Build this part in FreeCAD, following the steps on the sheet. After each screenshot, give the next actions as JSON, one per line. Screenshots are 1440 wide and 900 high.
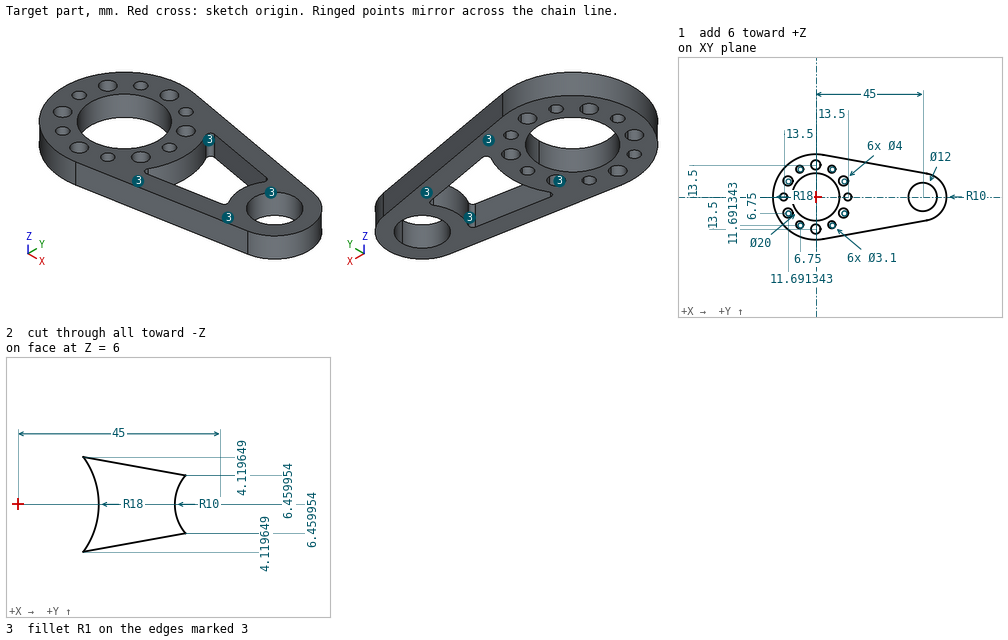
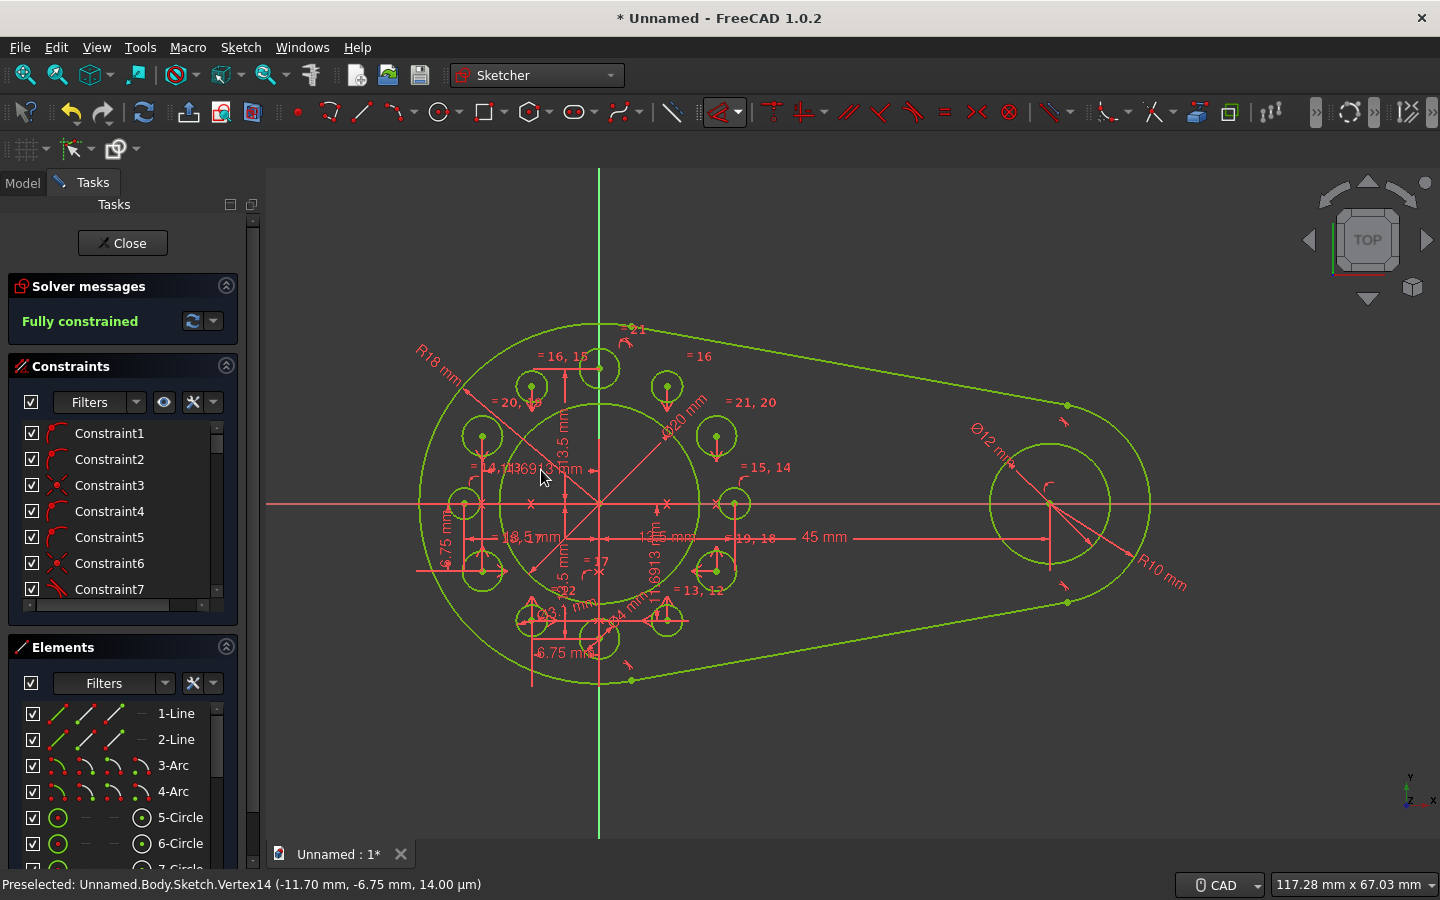
{"action": "left_click", "coordinate": [123, 243]}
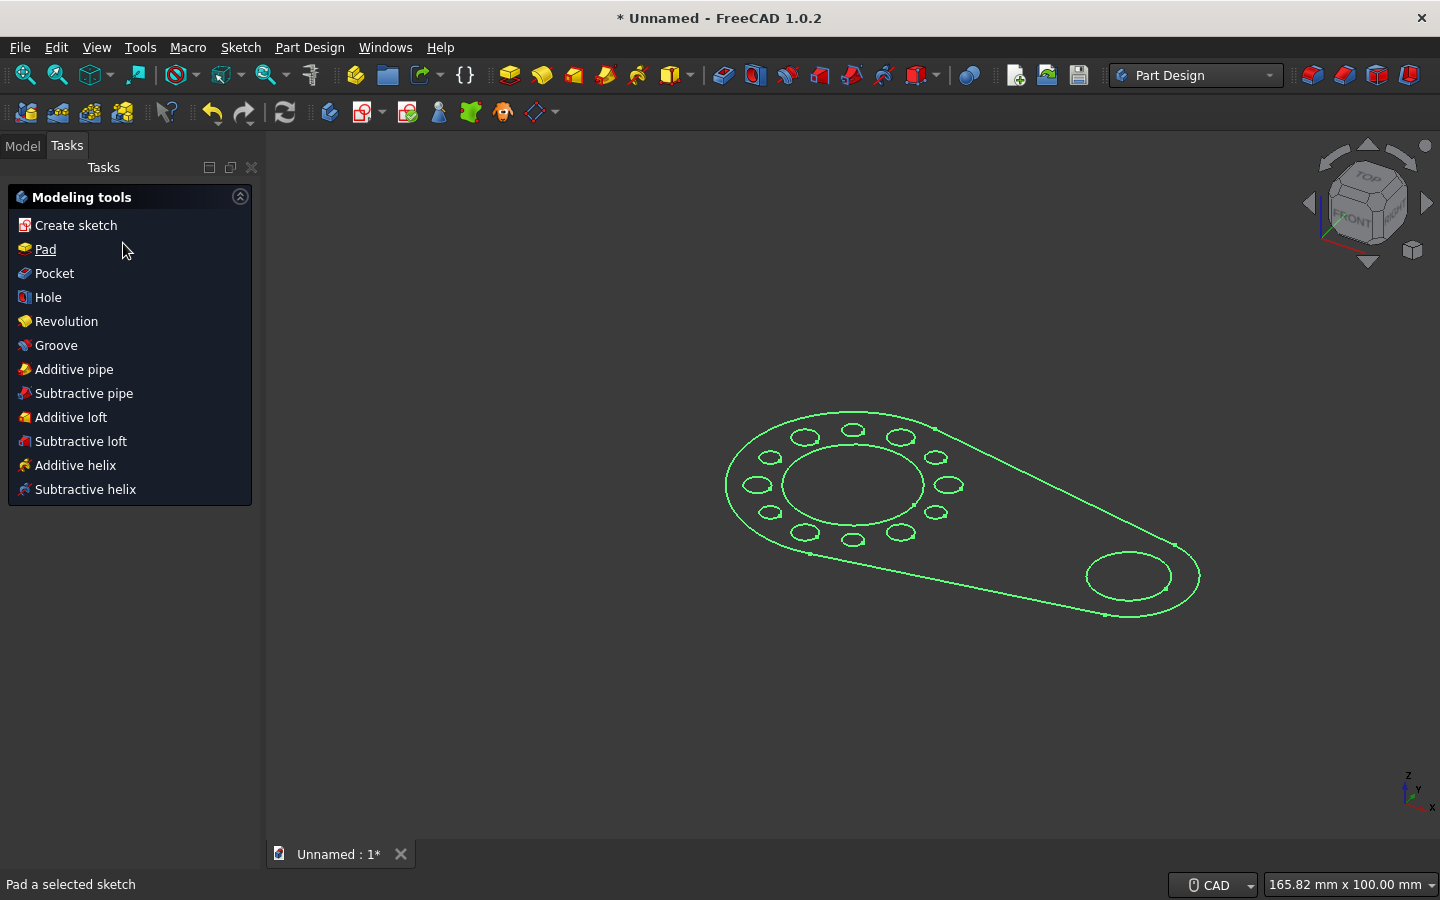
{"action": "left_click", "coordinate": [510, 76]}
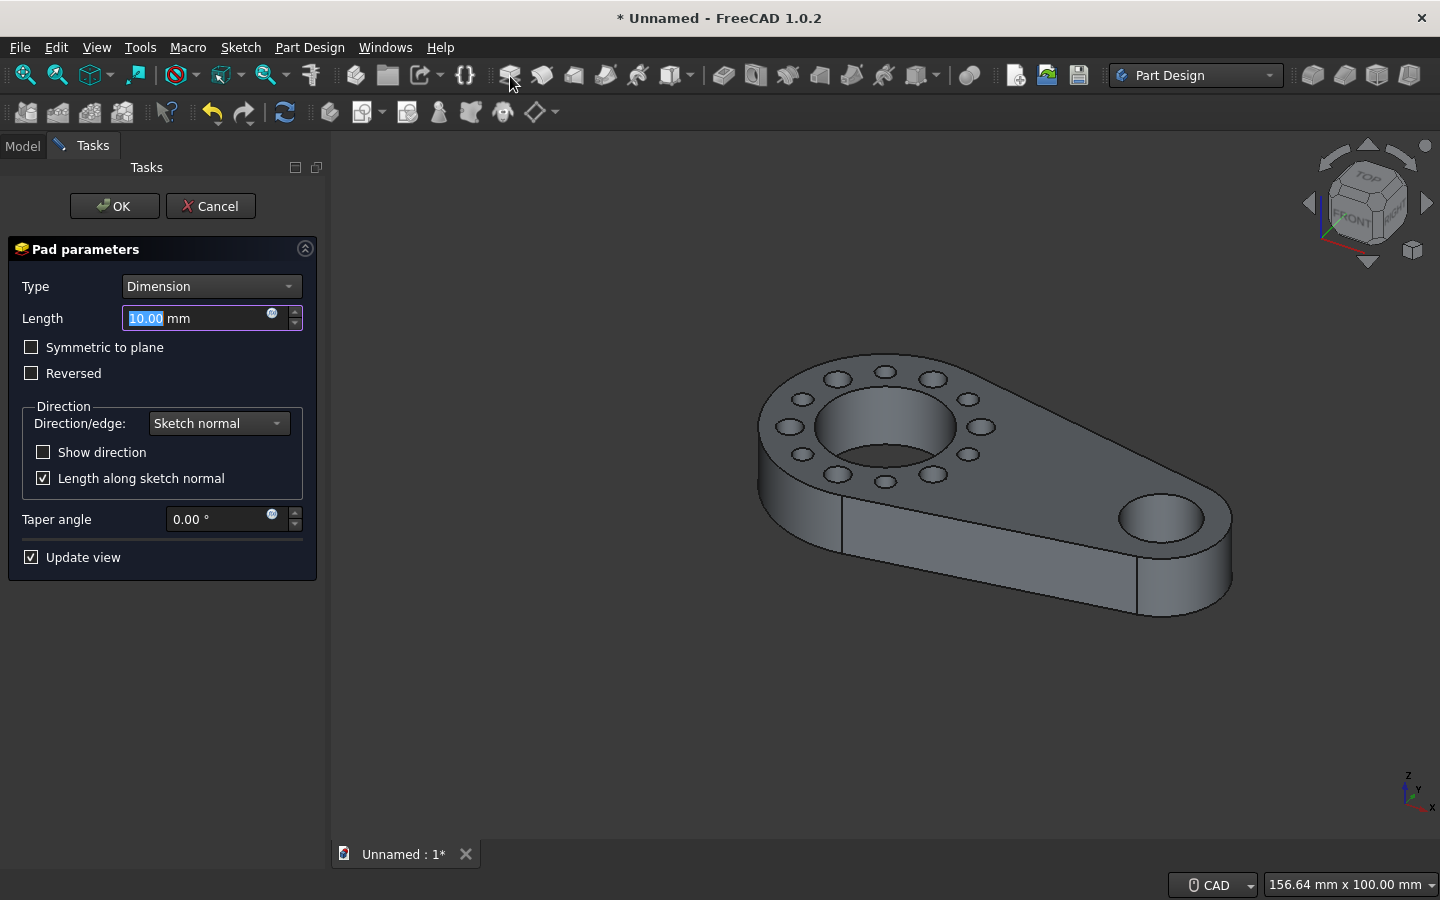
{"action": "type", "text": "6"}
{"action": "key", "text": "Tab"}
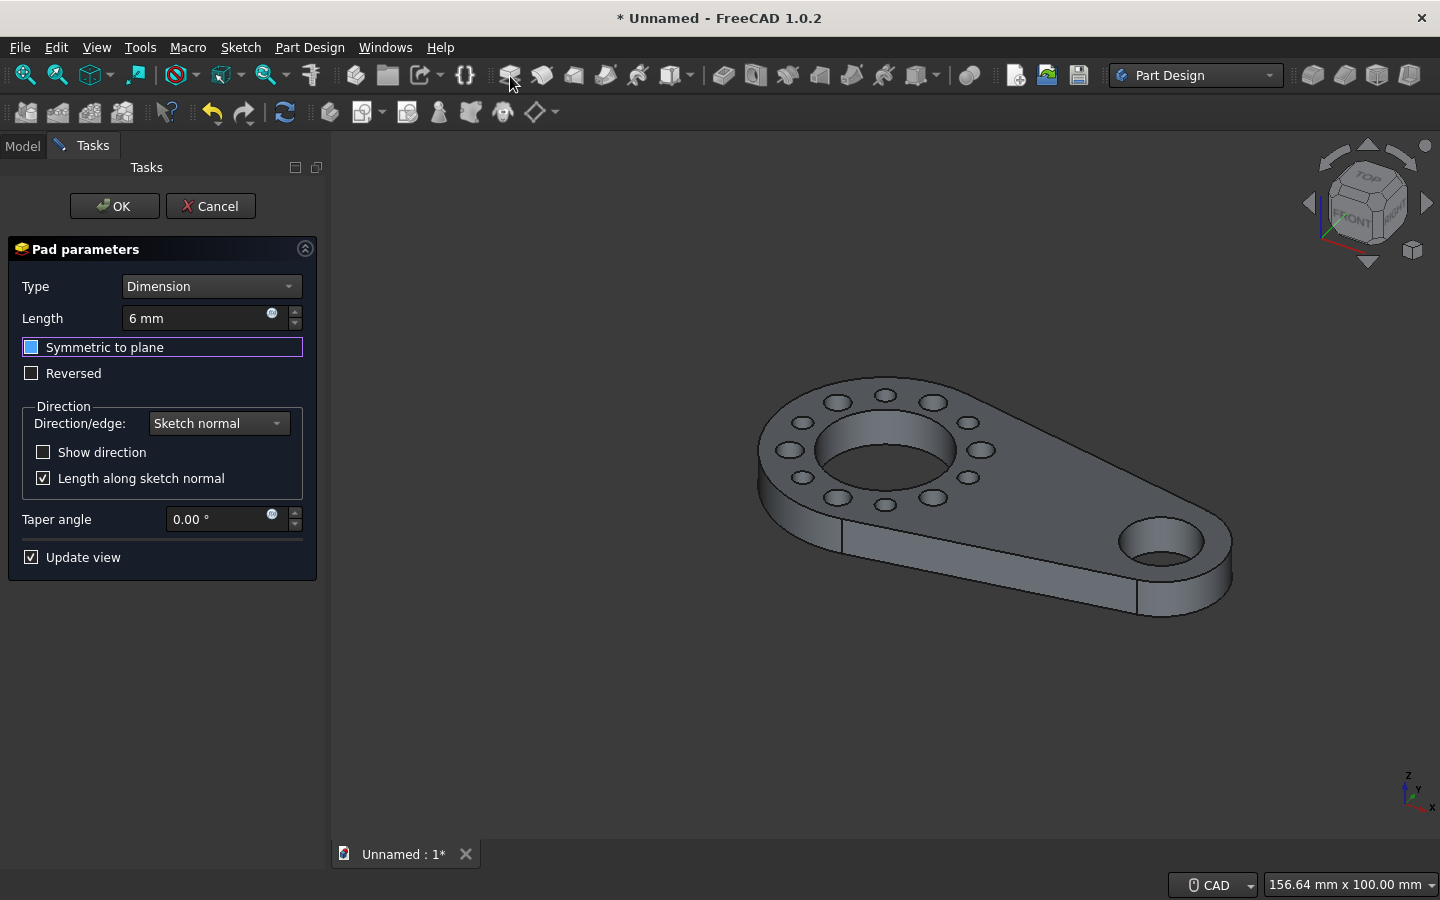
{"action": "left_click", "coordinate": [115, 206]}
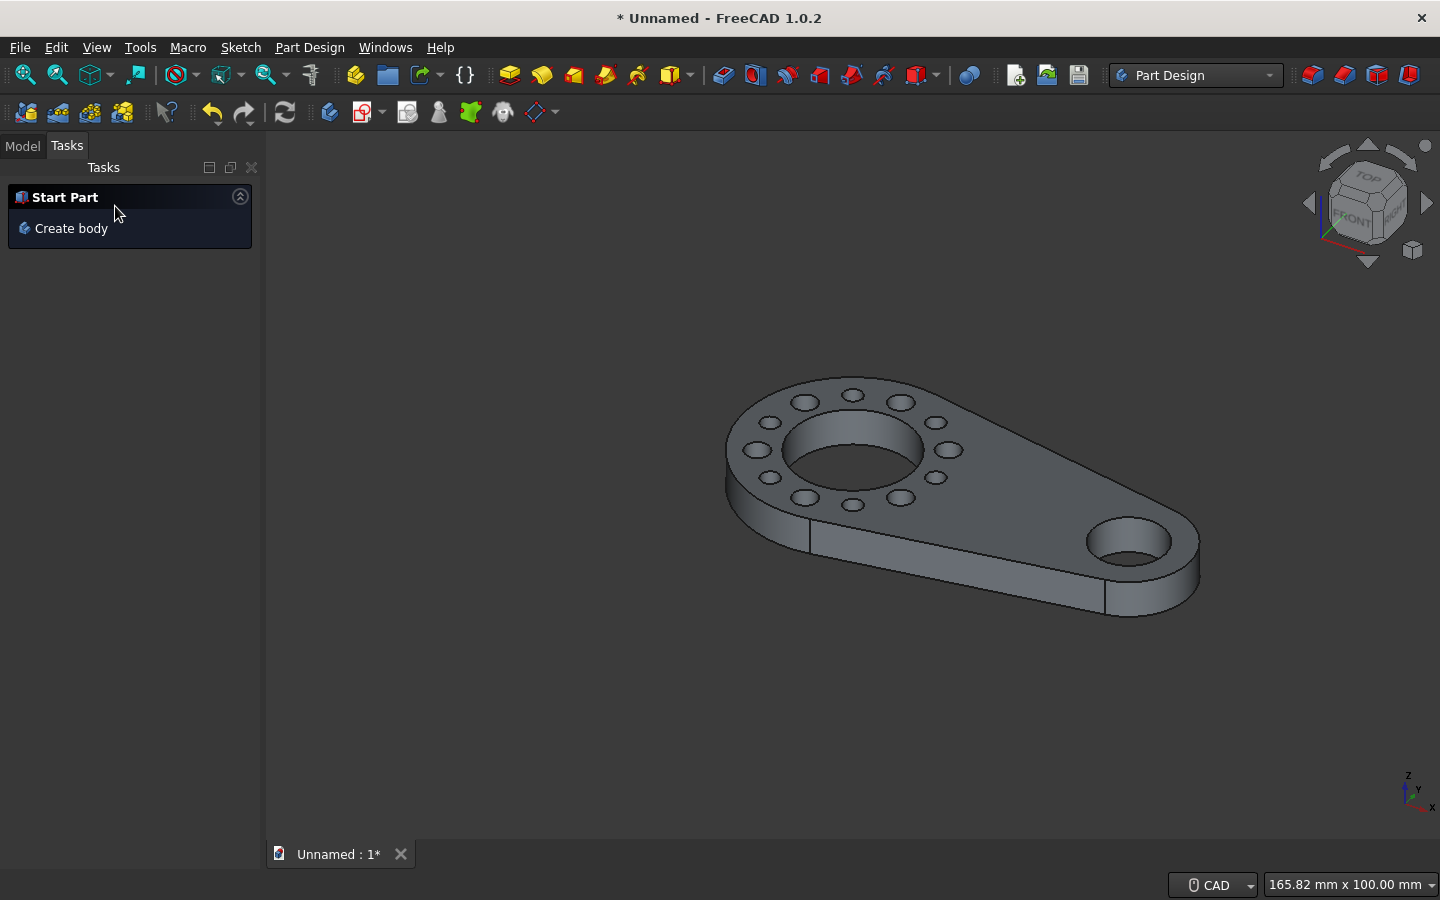
{"action": "left_click", "coordinate": [1030, 508]}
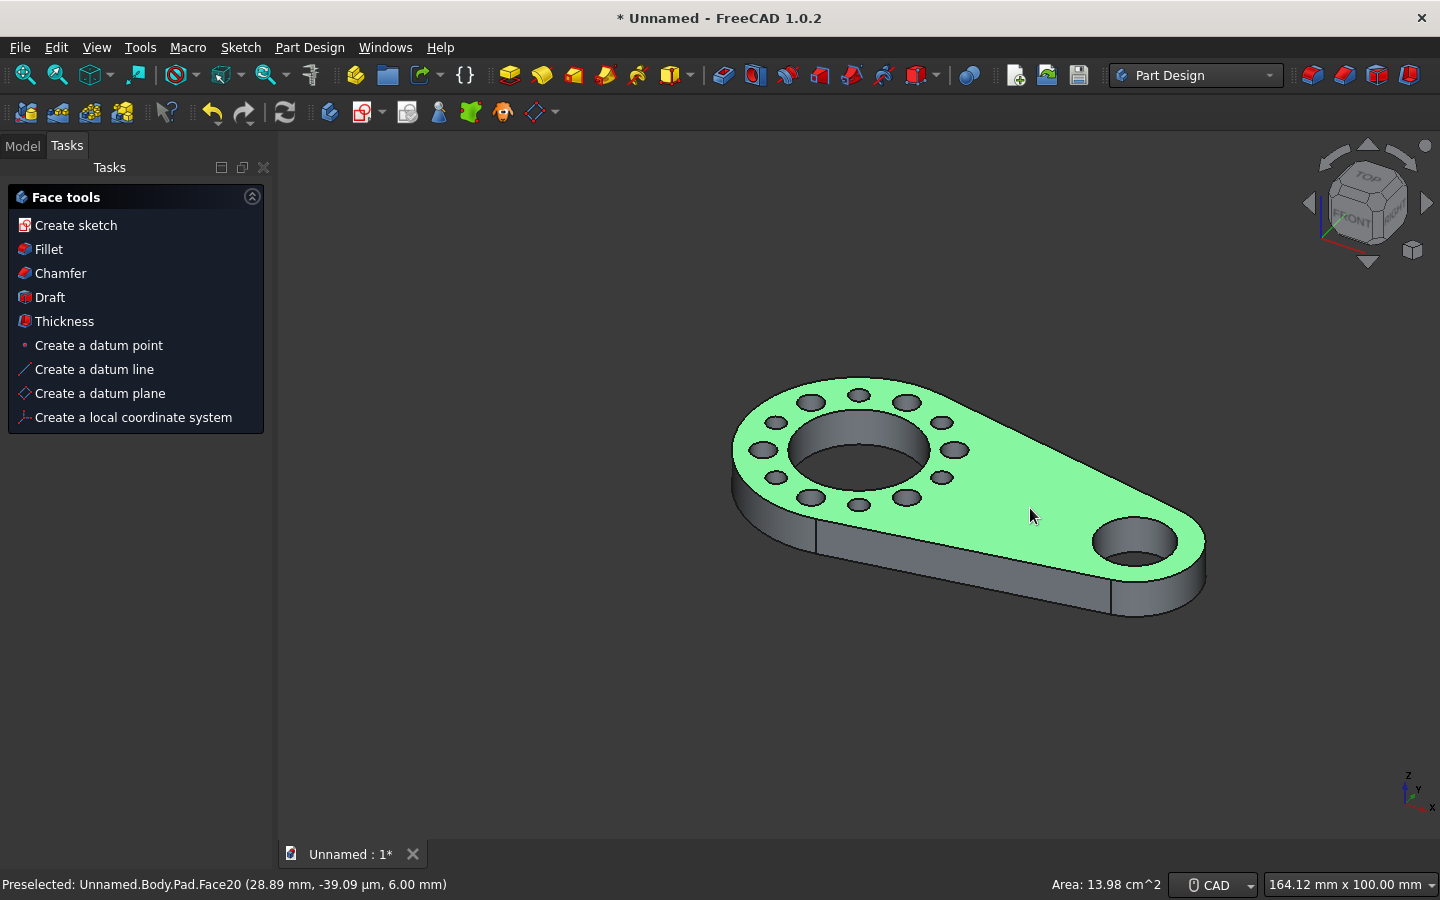
{"action": "left_click", "coordinate": [362, 112]}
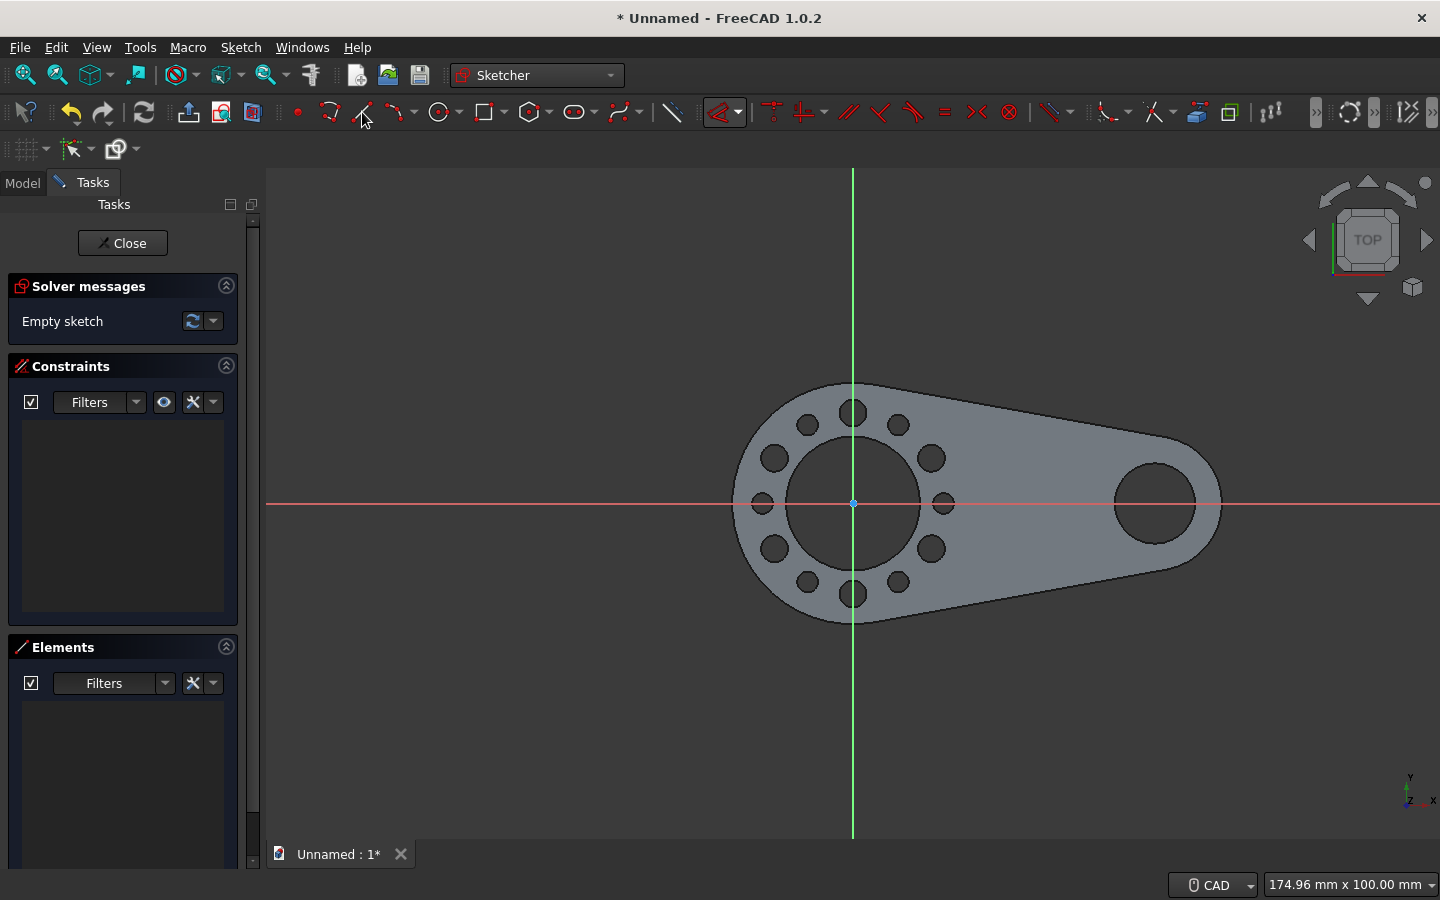
{"action": "scroll", "coordinate": [1091, 504], "scroll_direction": "up", "scroll_amount": 5}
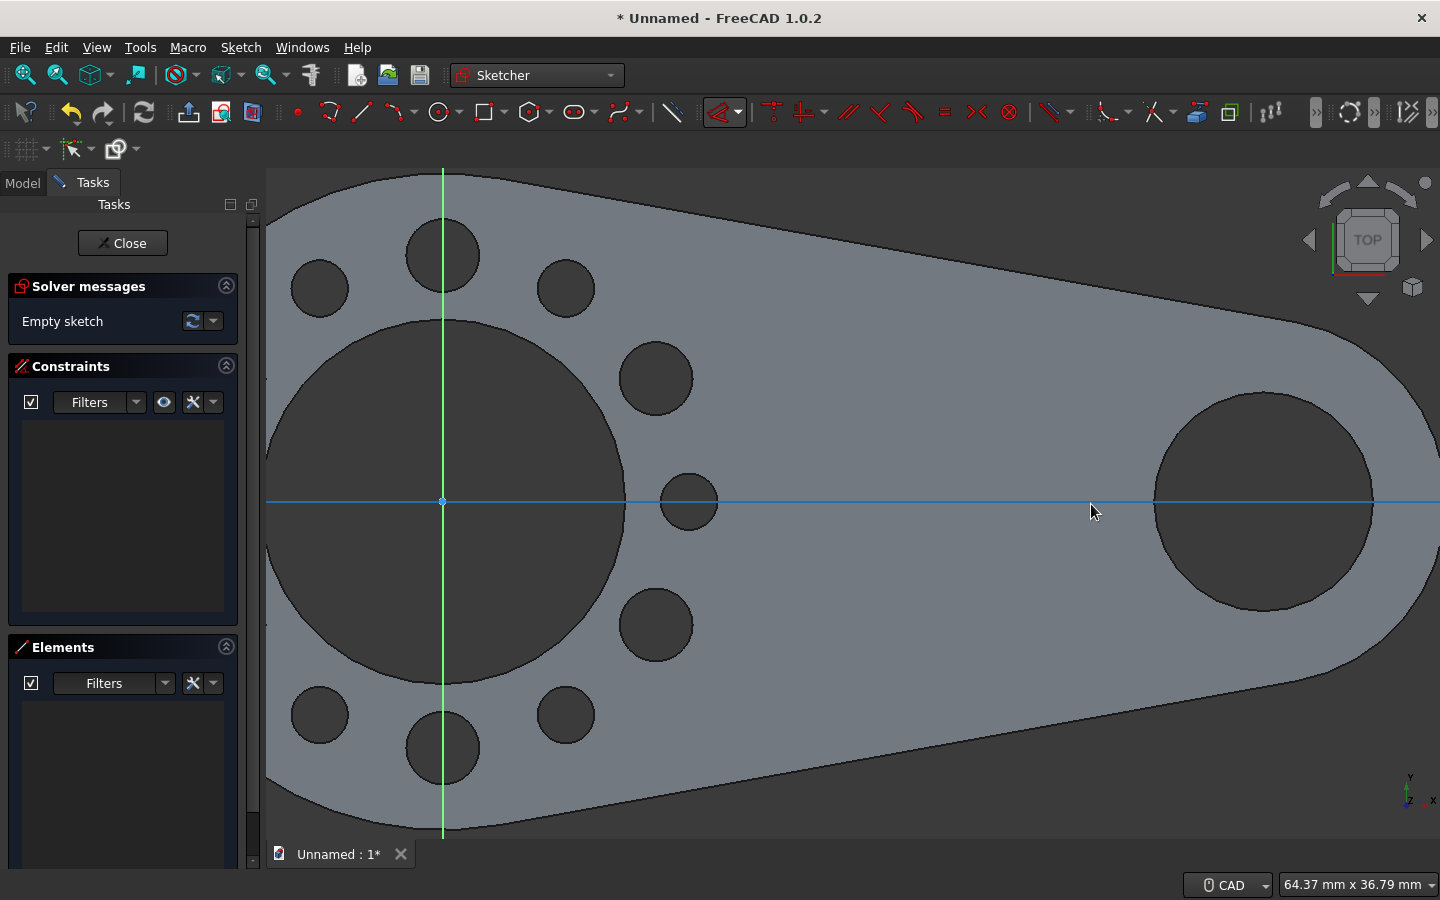
{"action": "key", "text": "g l"}